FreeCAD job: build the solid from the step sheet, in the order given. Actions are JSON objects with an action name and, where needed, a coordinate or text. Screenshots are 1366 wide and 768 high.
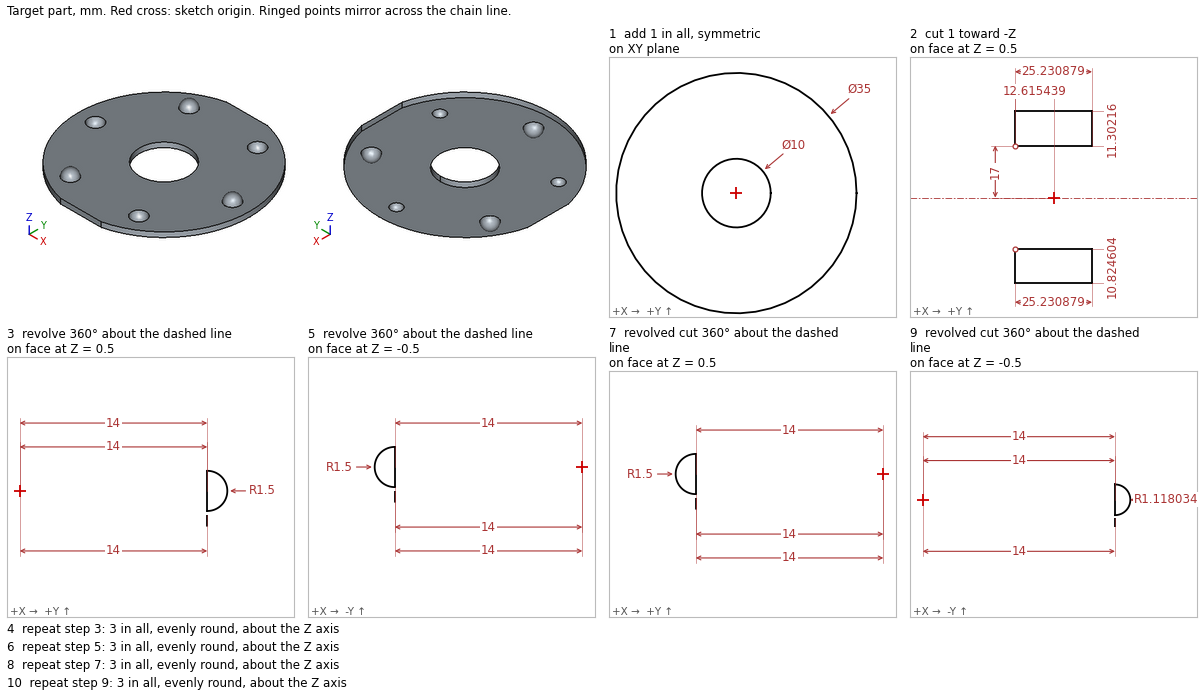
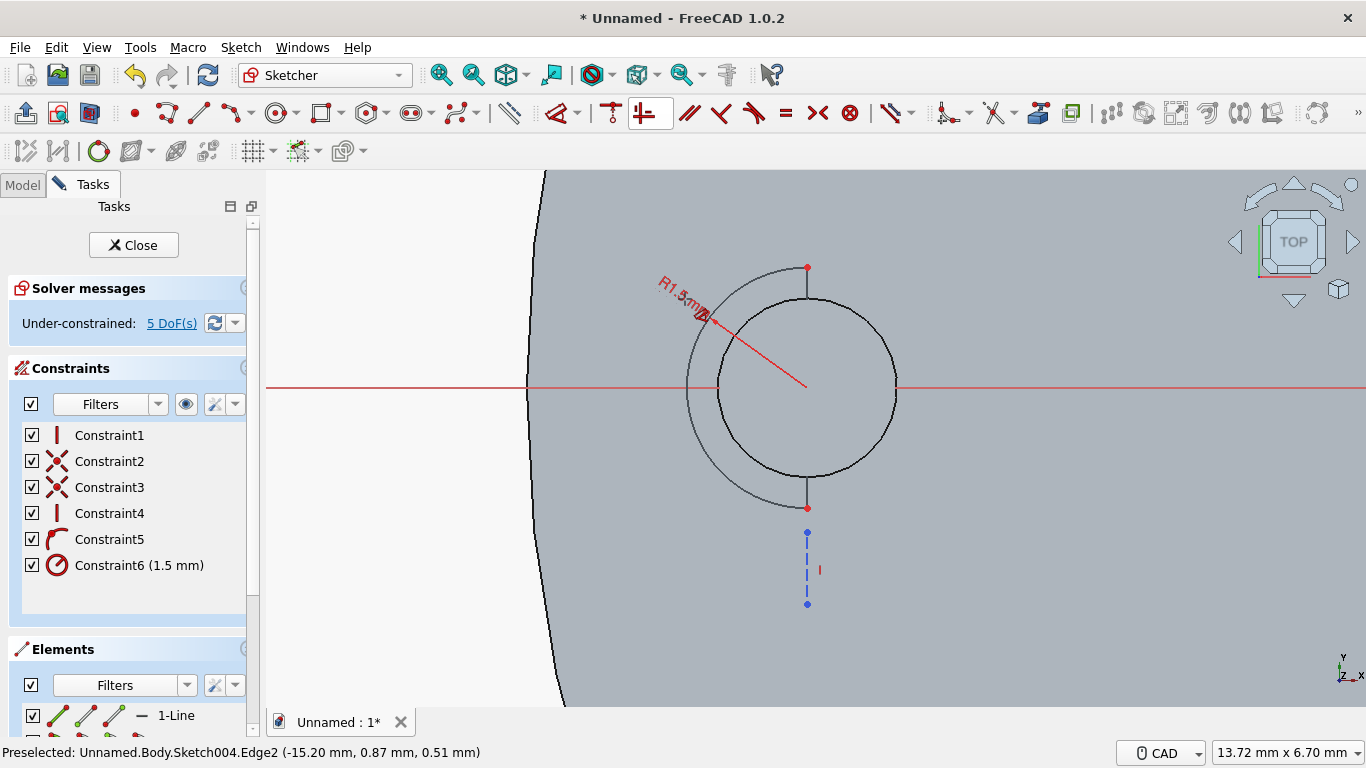
{"action": "left_click", "coordinate": [807, 508]}
{"action": "left_click", "coordinate": [1004, 542]}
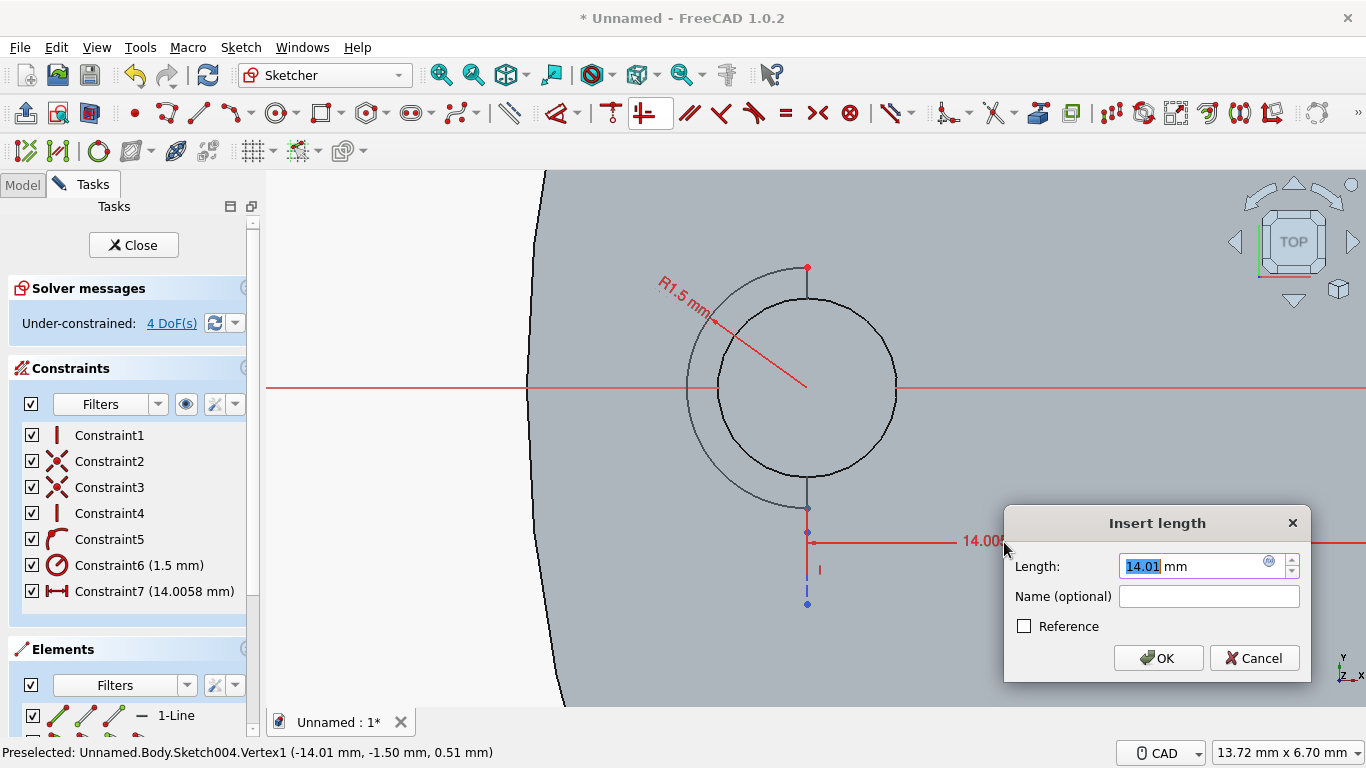
{"action": "type", "text": "14"}
{"action": "key", "text": "Return"}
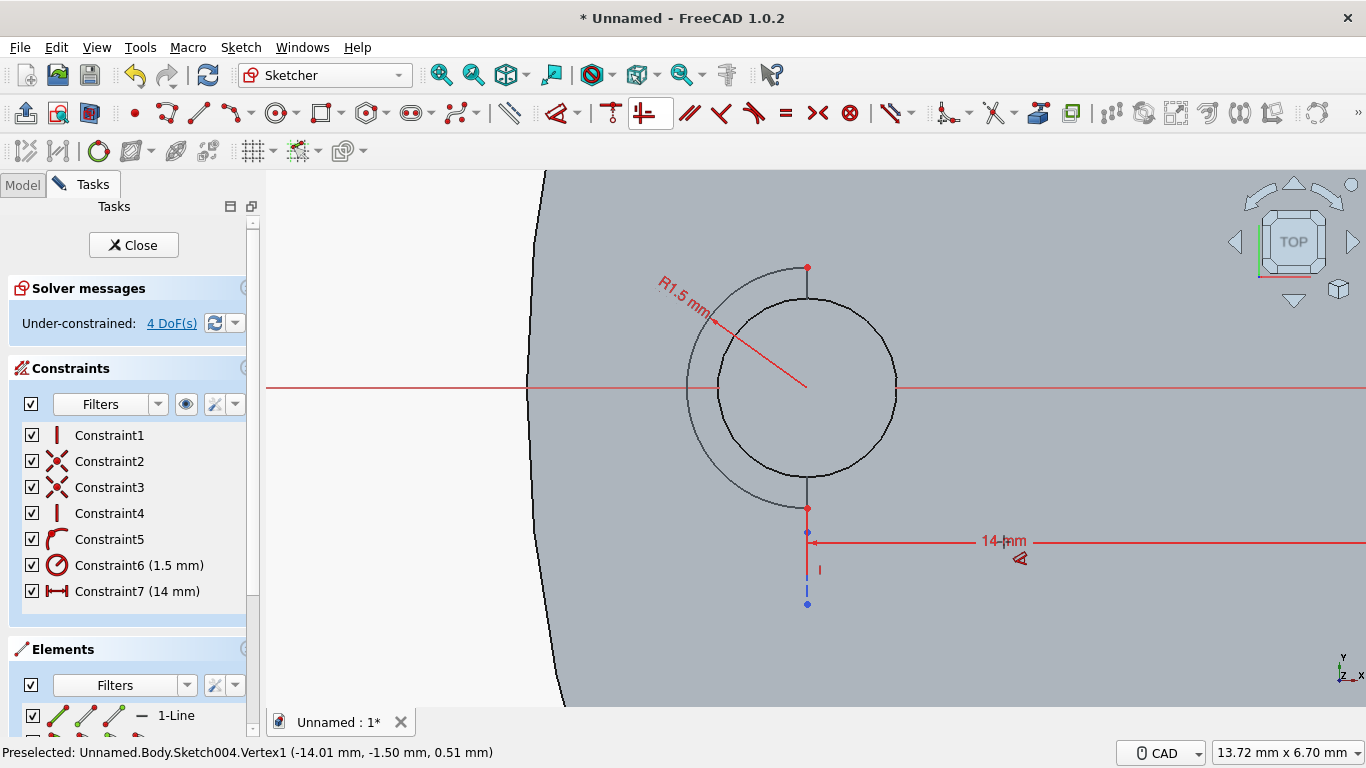
{"action": "left_click", "coordinate": [807, 533]}
{"action": "left_click", "coordinate": [1004, 567]}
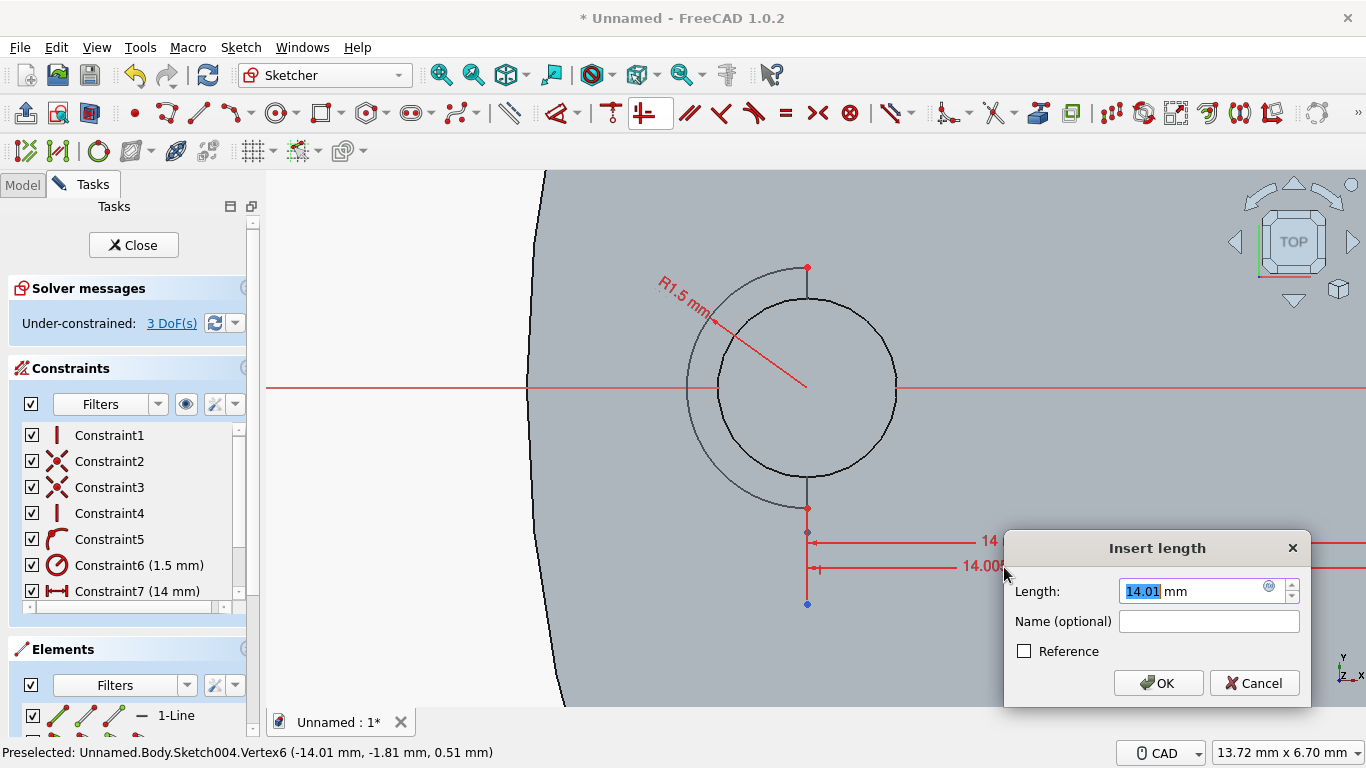
{"action": "type", "text": "14"}
{"action": "key", "text": "Return"}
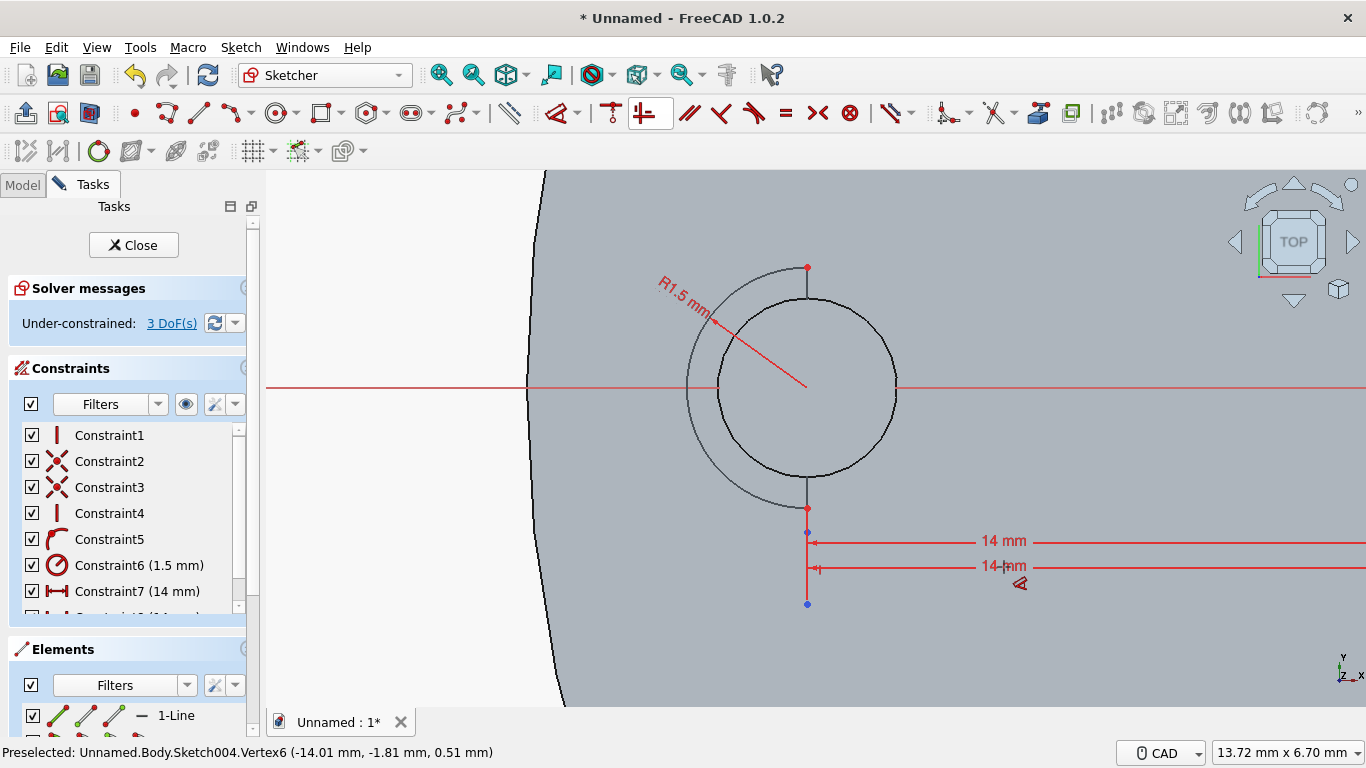
{"action": "left_click", "coordinate": [807, 388]}
{"action": "left_click", "coordinate": [1004, 354]}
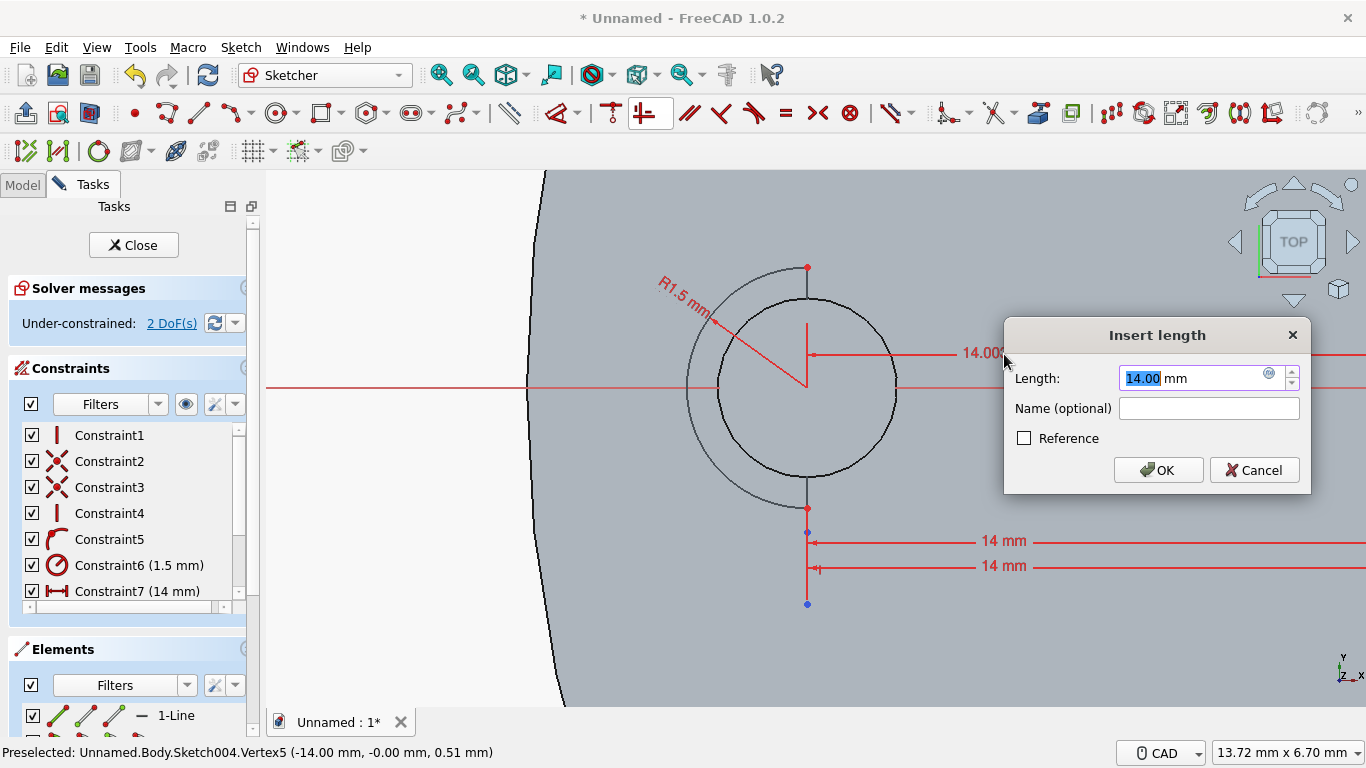
{"action": "type", "text": "14"}
{"action": "key", "text": "Return"}
{"action": "key", "text": "Escape"}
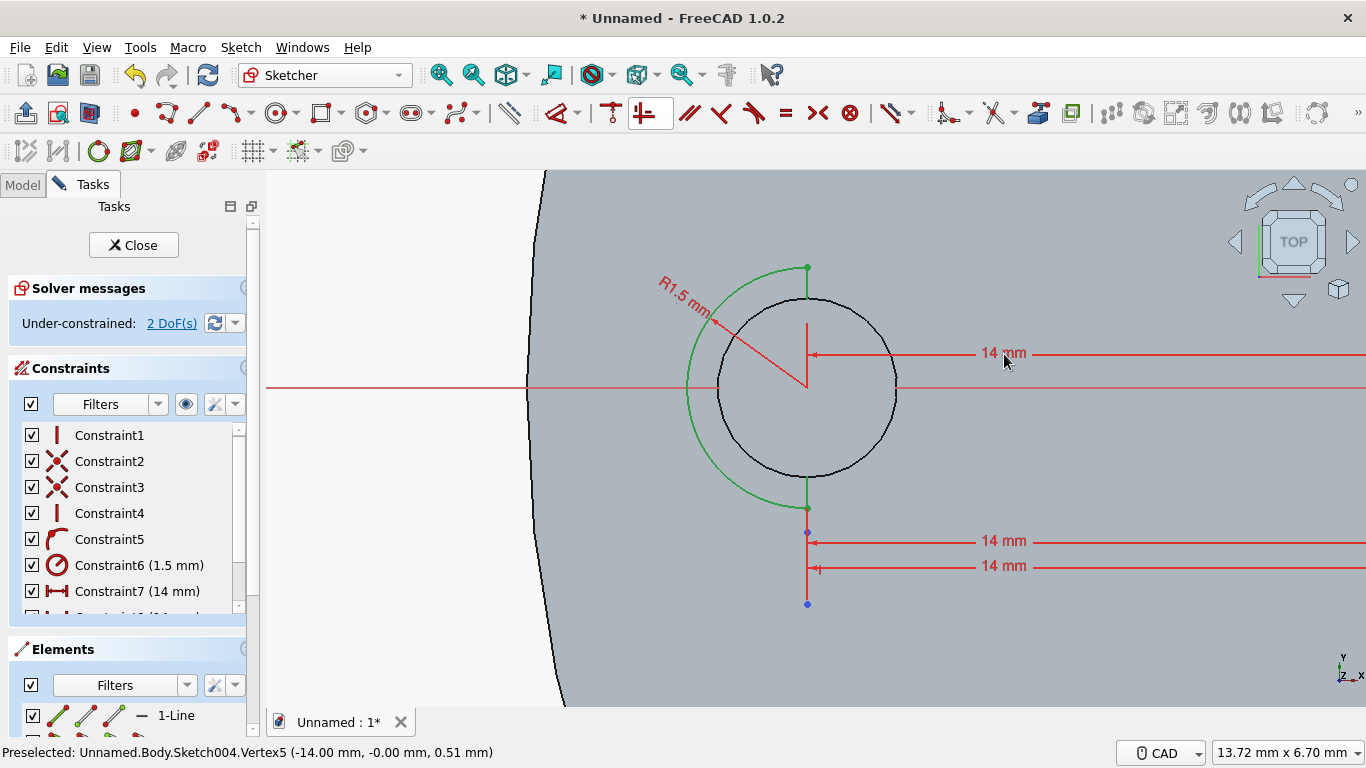
{"action": "left_click", "coordinate": [134, 245]}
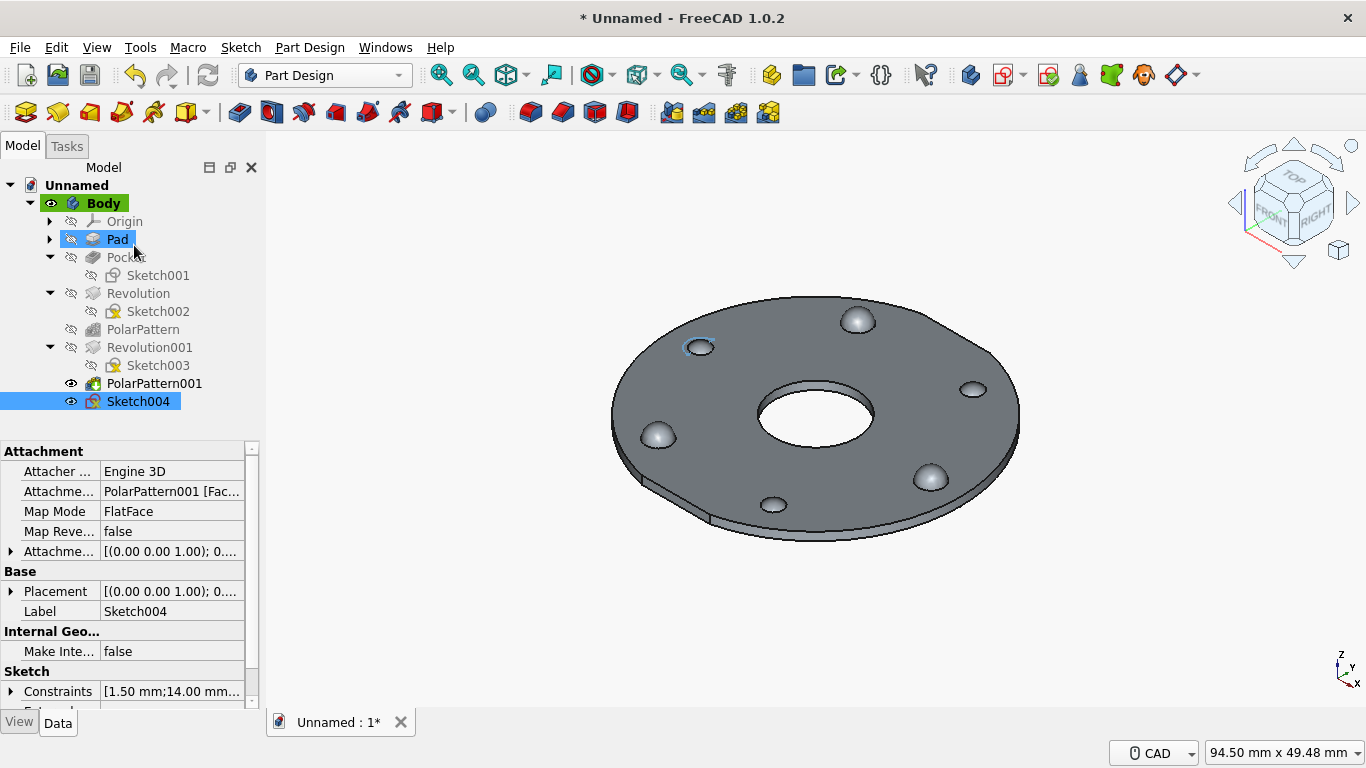
{"action": "left_click", "coordinate": [304, 112]}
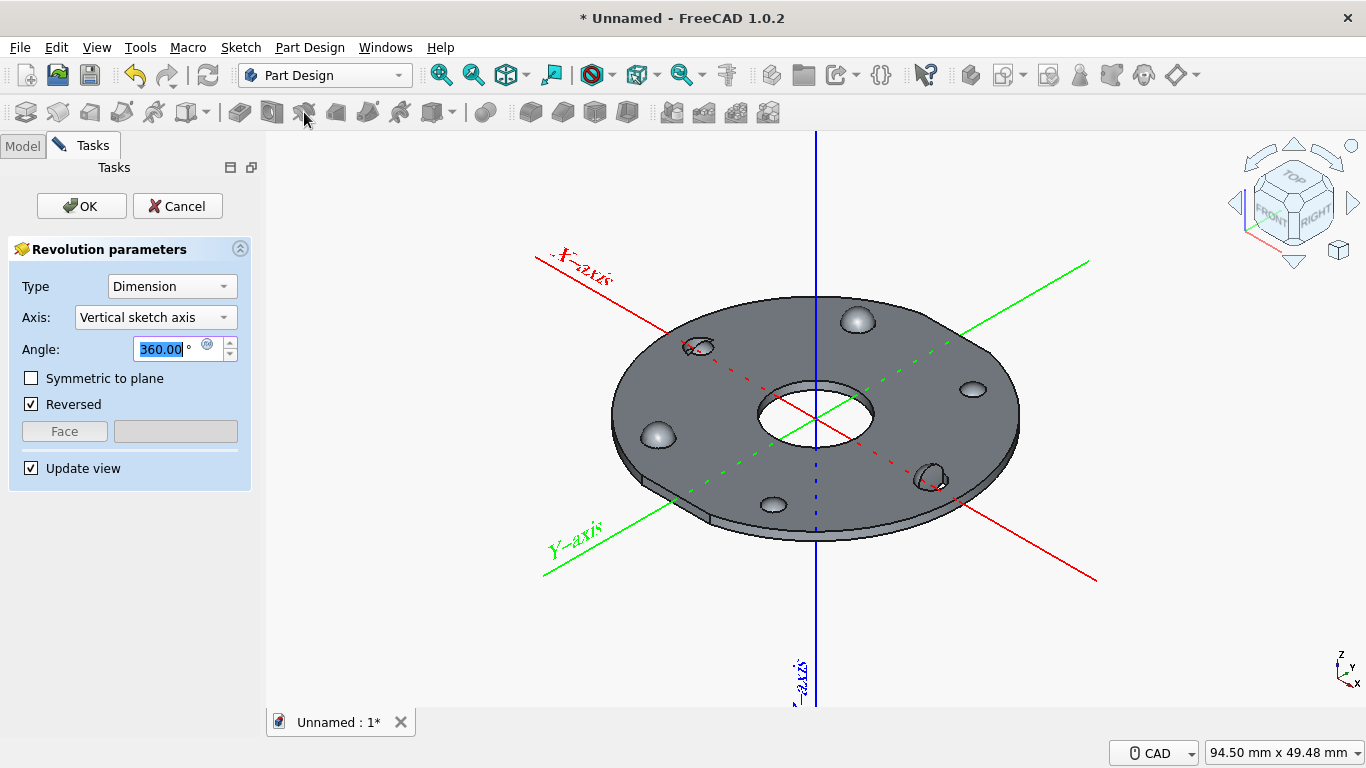
{"action": "left_click", "coordinate": [156, 318]}